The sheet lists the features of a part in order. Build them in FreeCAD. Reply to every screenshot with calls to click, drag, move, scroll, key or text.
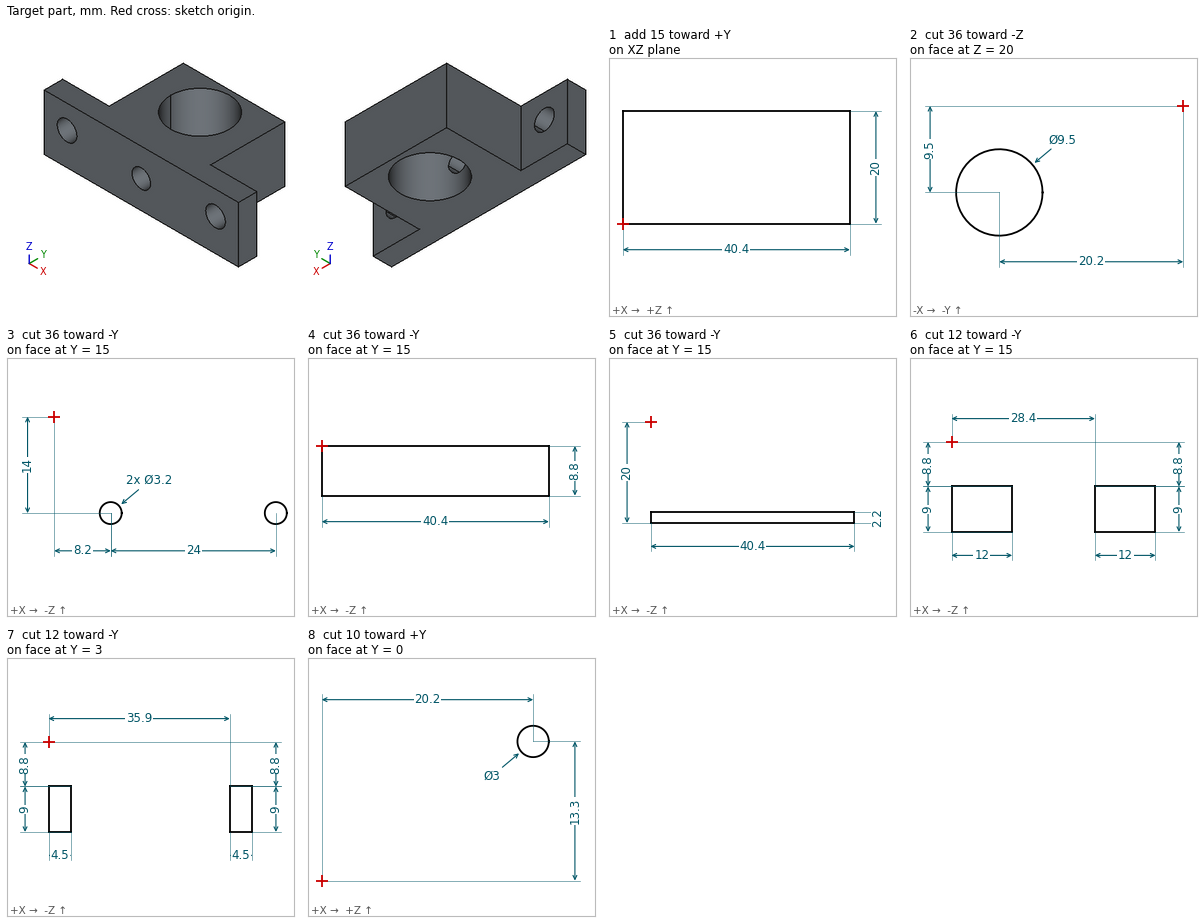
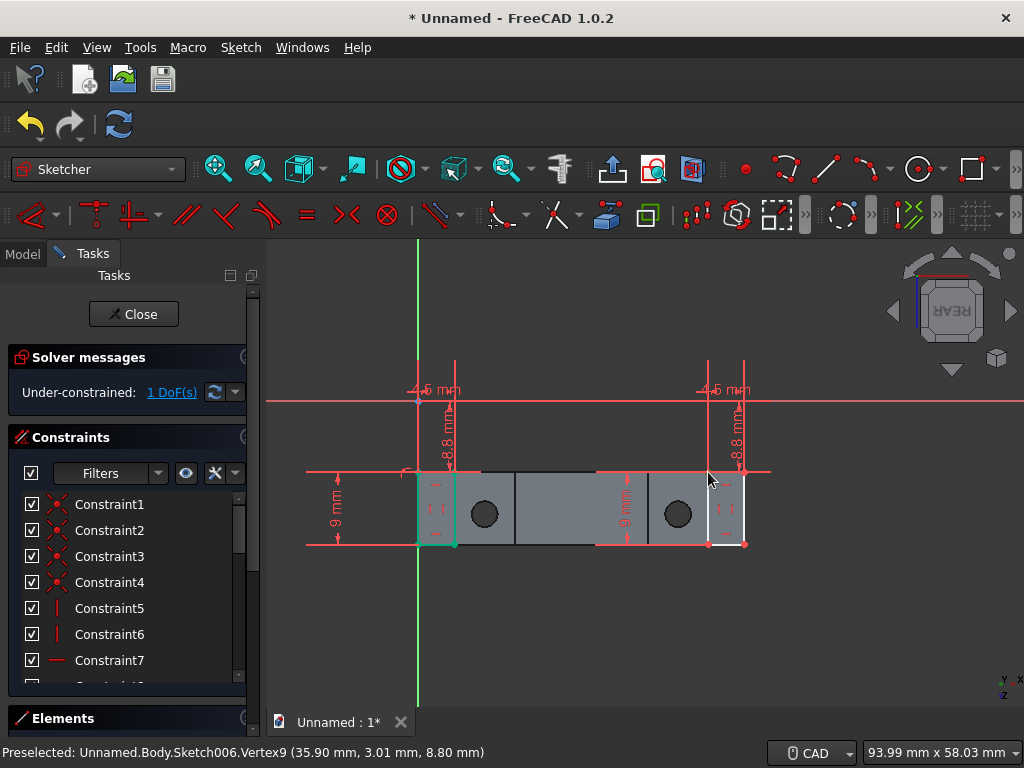
key(l)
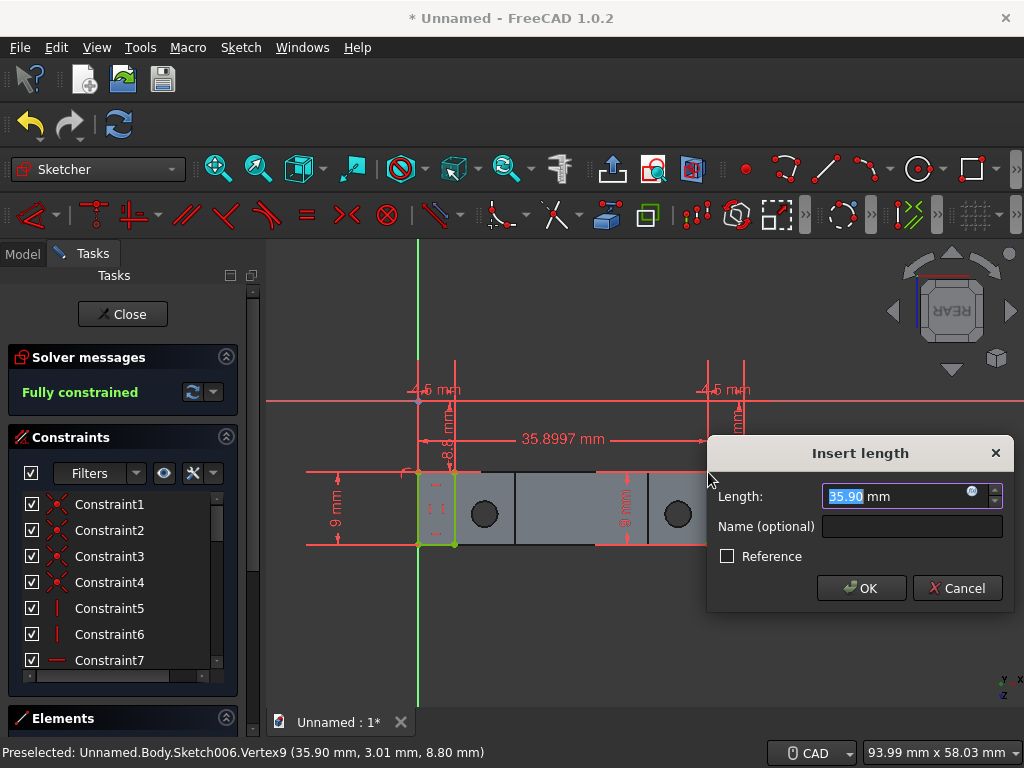
text(35.9)
key(Return)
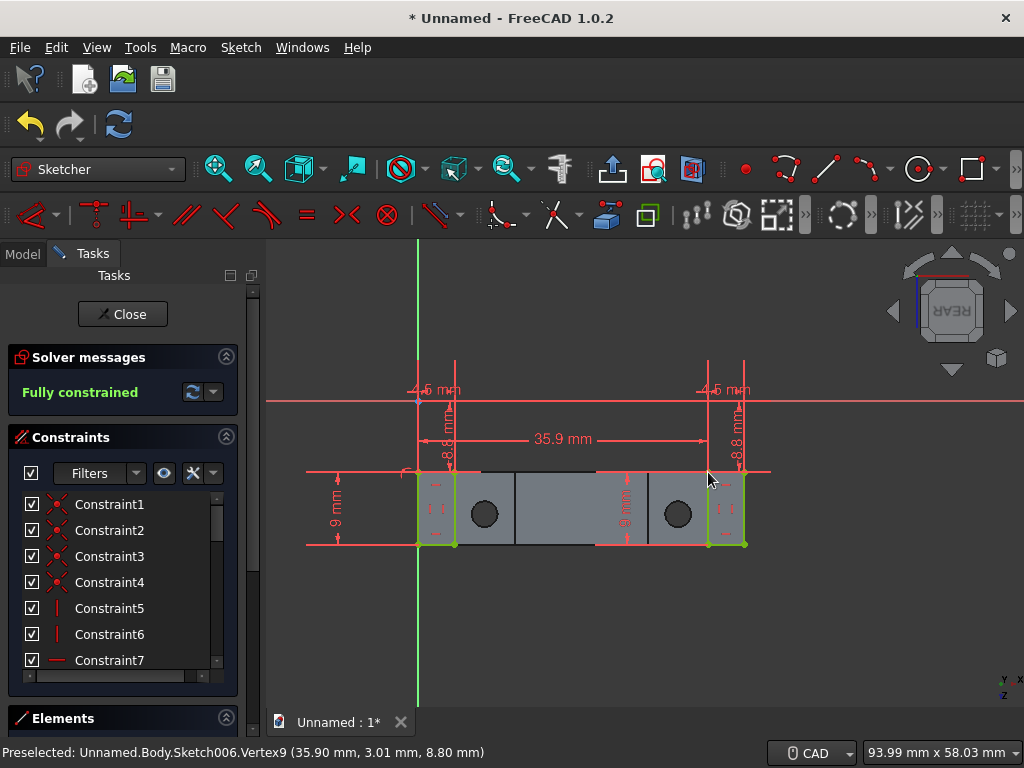
click(123, 314)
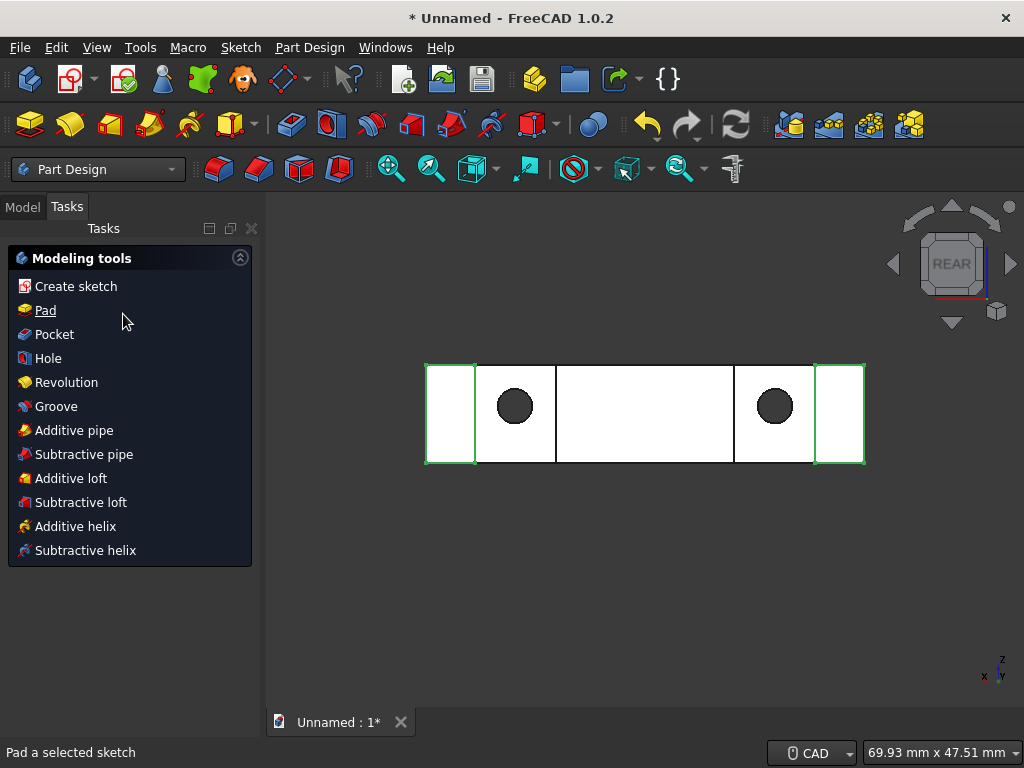
click(292, 124)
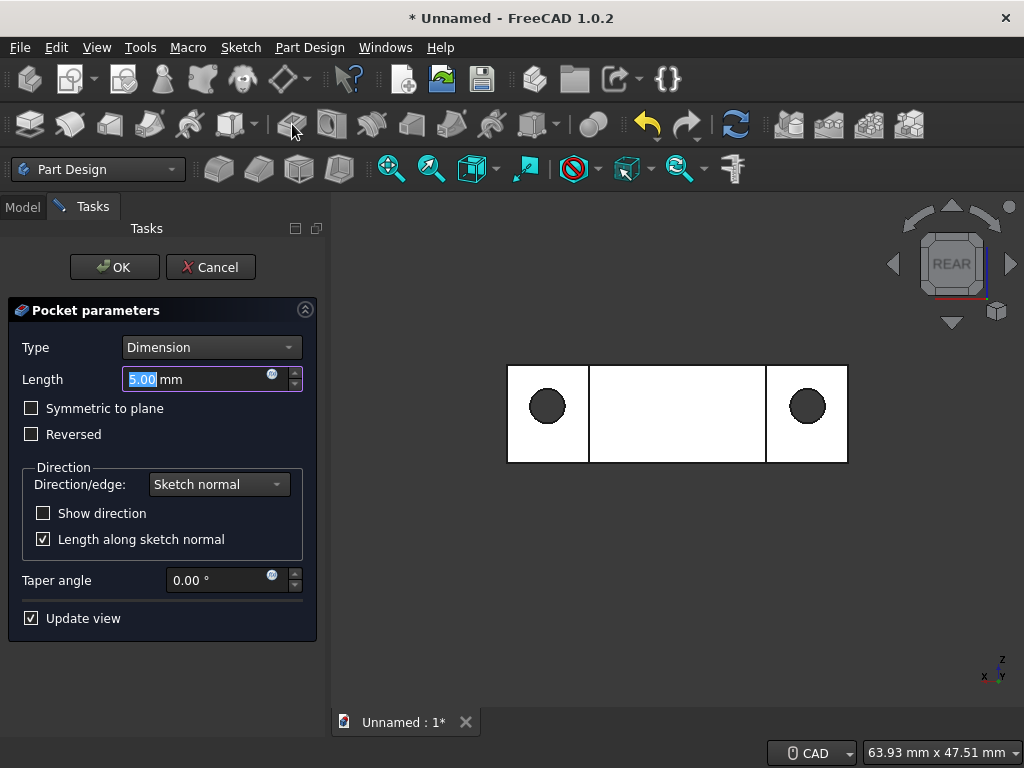
text(12)
key(Tab)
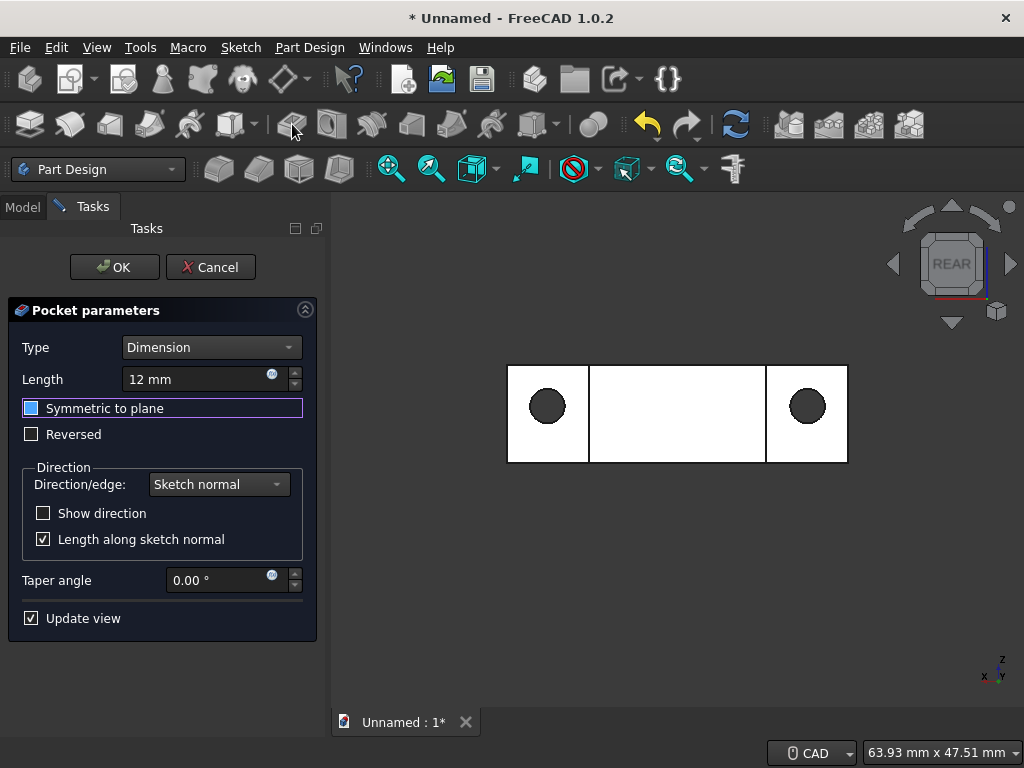
click(115, 267)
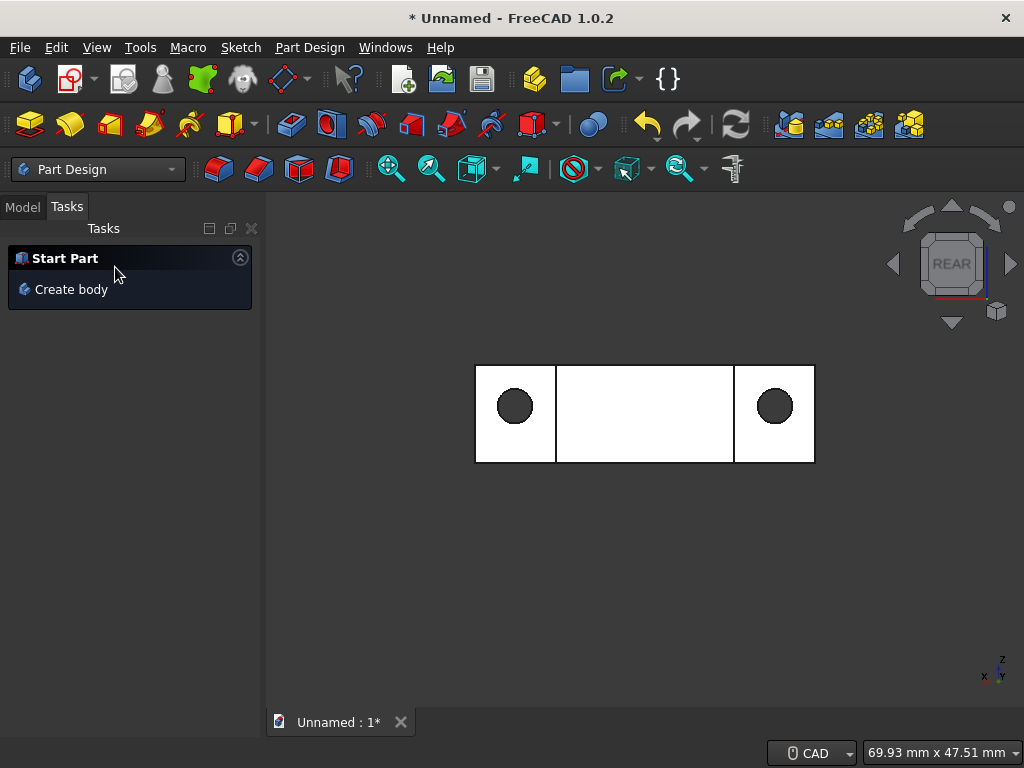
click(392, 170)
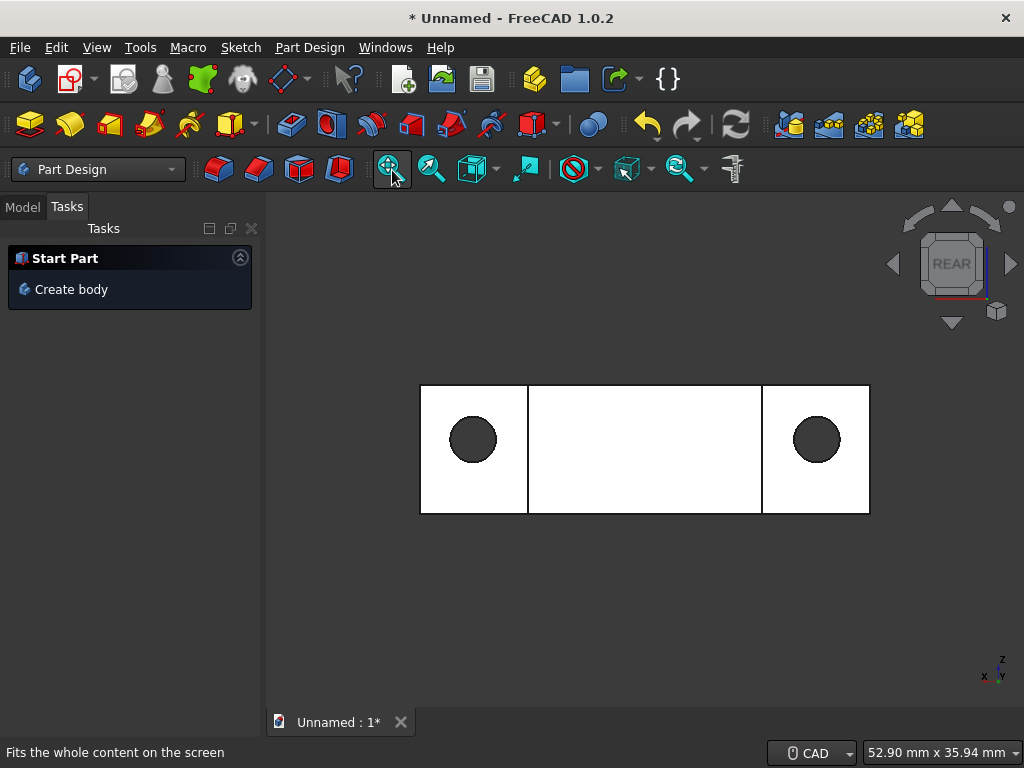
key(0)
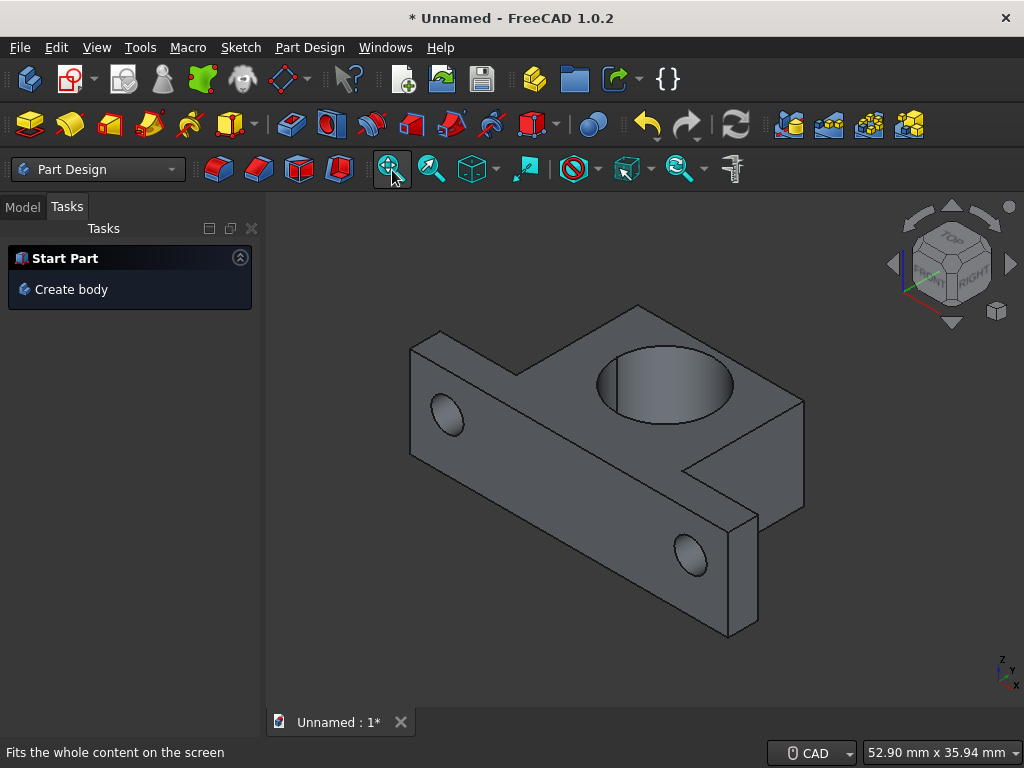
click(614, 519)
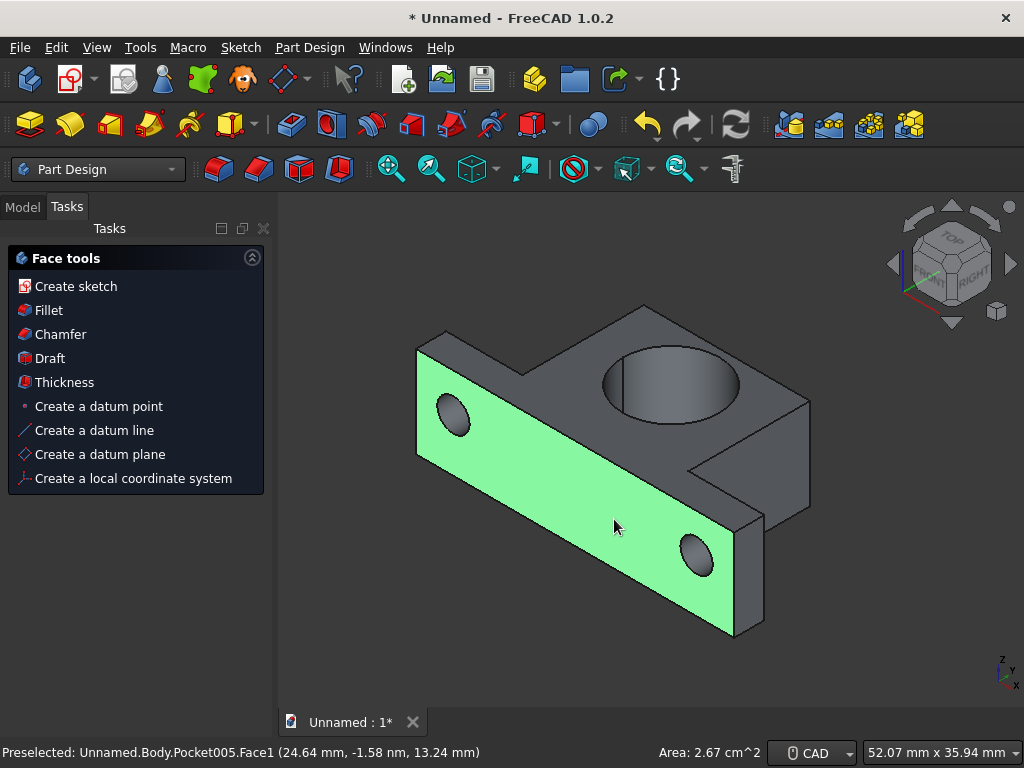
click(70, 80)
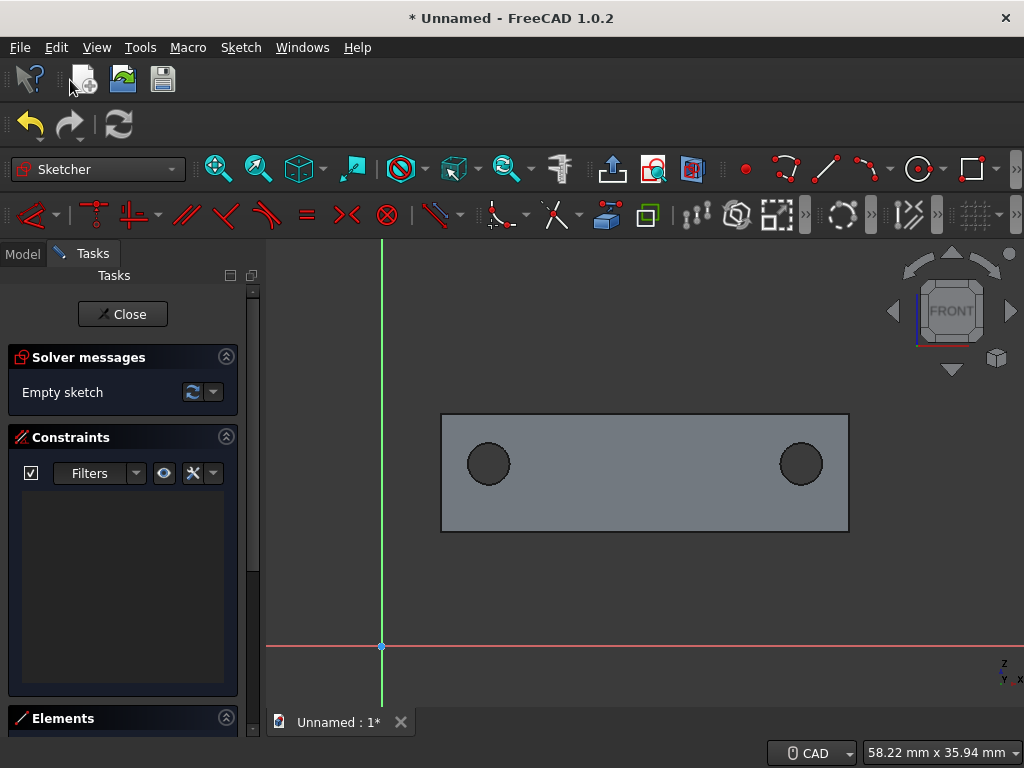
scroll(656, 473, up, 10)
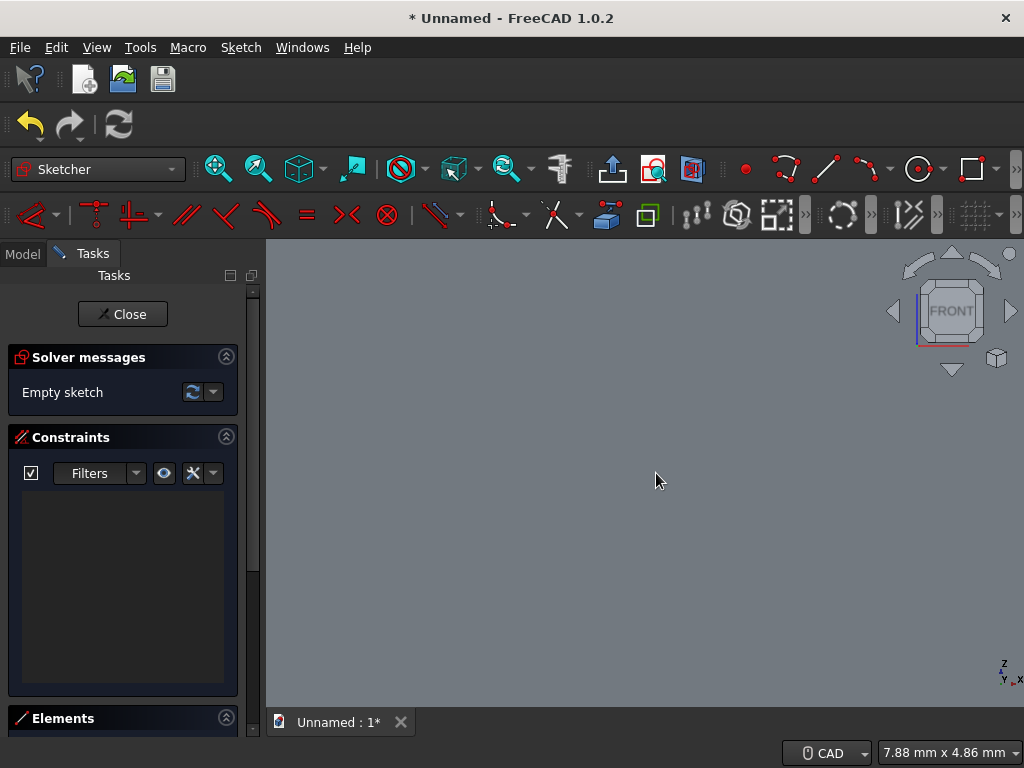
key(g)
key(c)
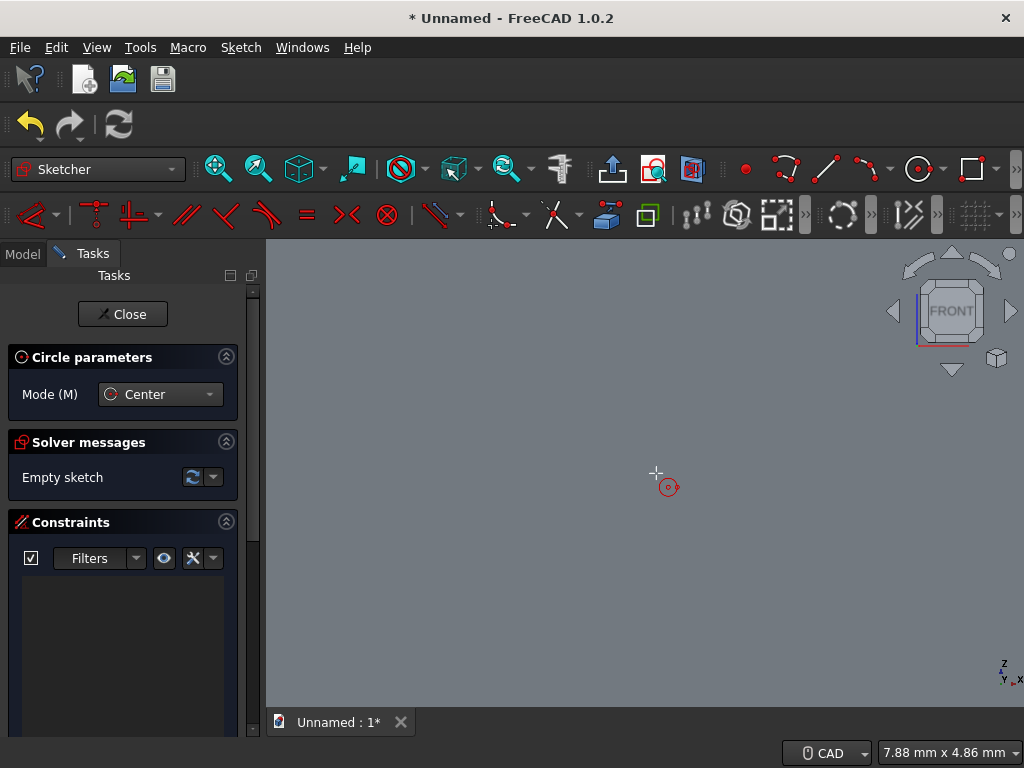
click(571, 470)
move(673, 368)